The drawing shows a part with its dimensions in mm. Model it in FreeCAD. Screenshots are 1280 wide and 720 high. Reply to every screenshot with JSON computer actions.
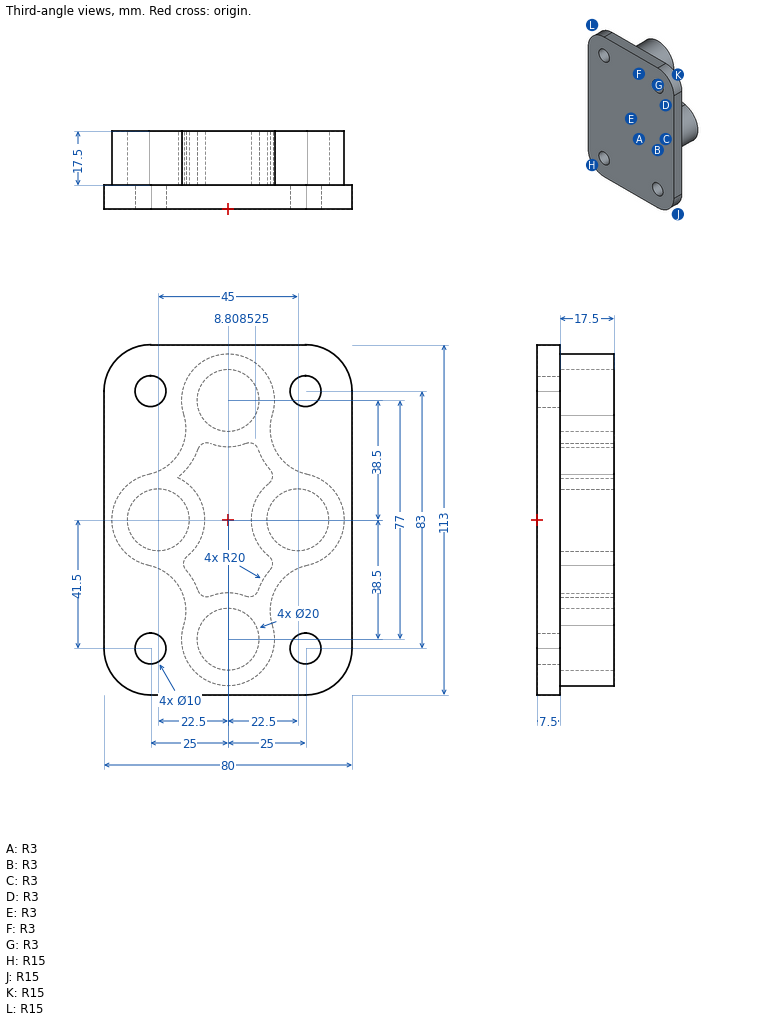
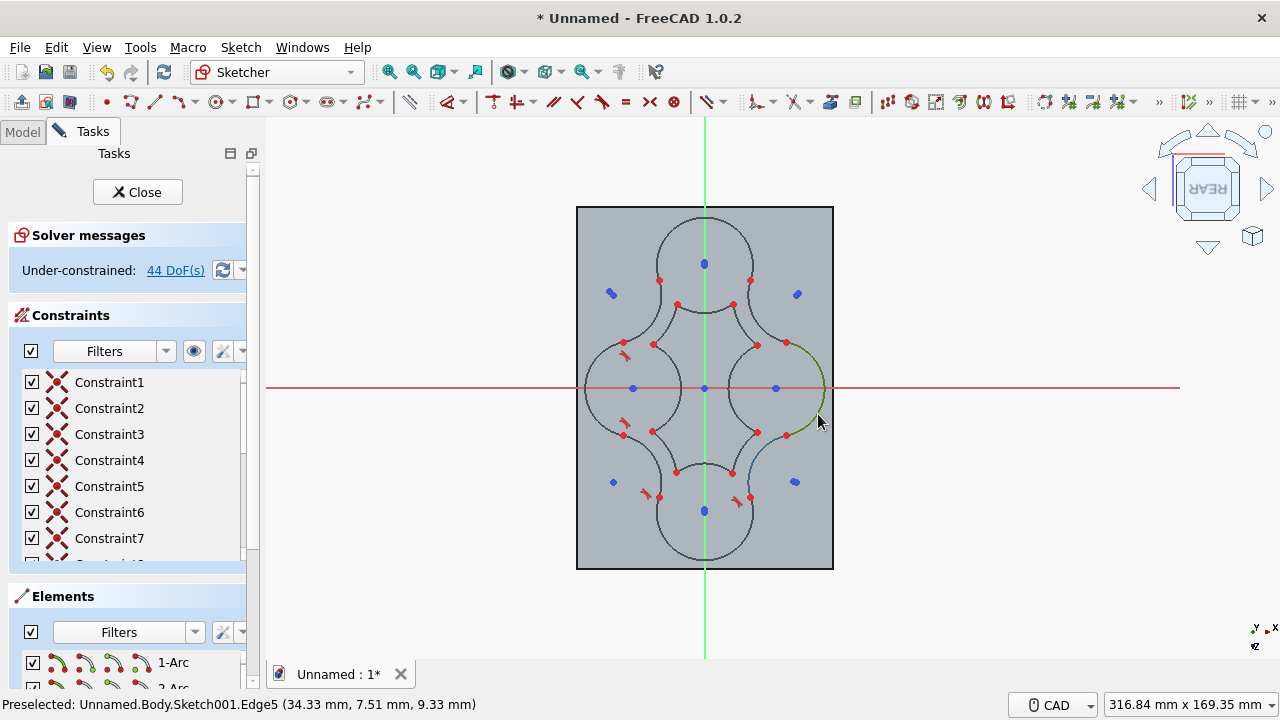
{"action": "key", "text": "t"}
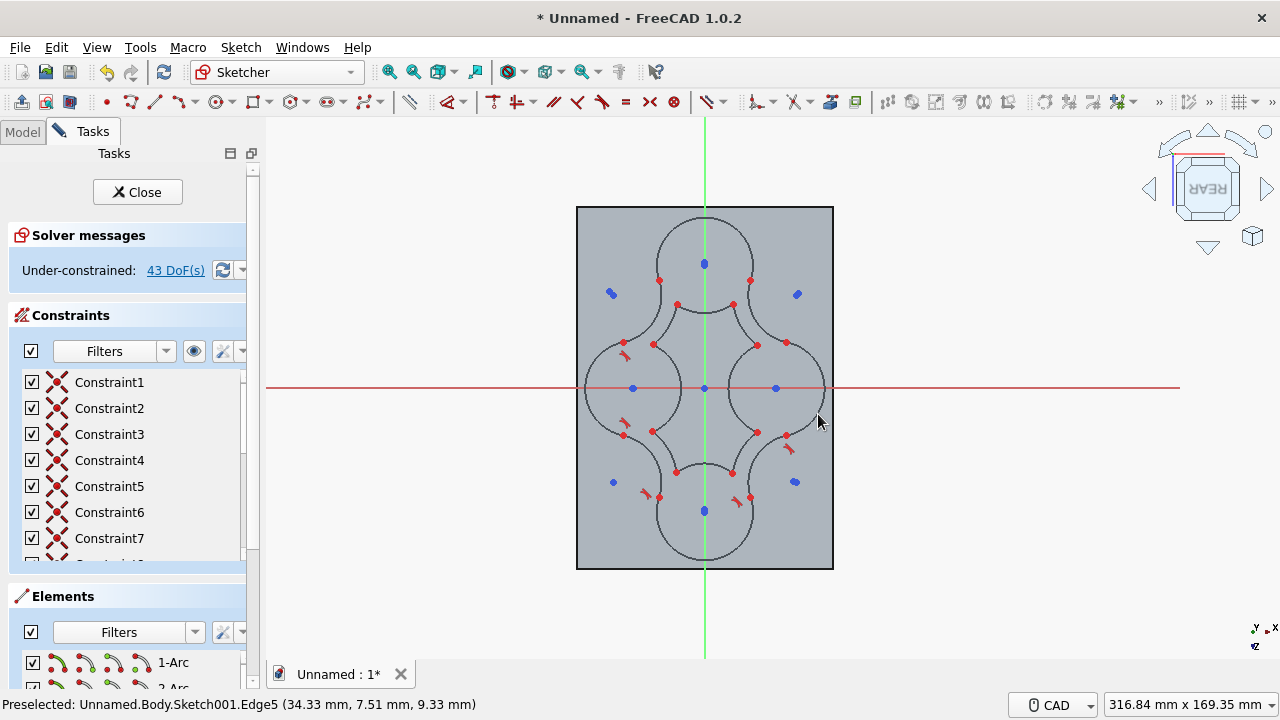
{"action": "left_click", "coordinate": [818, 414]}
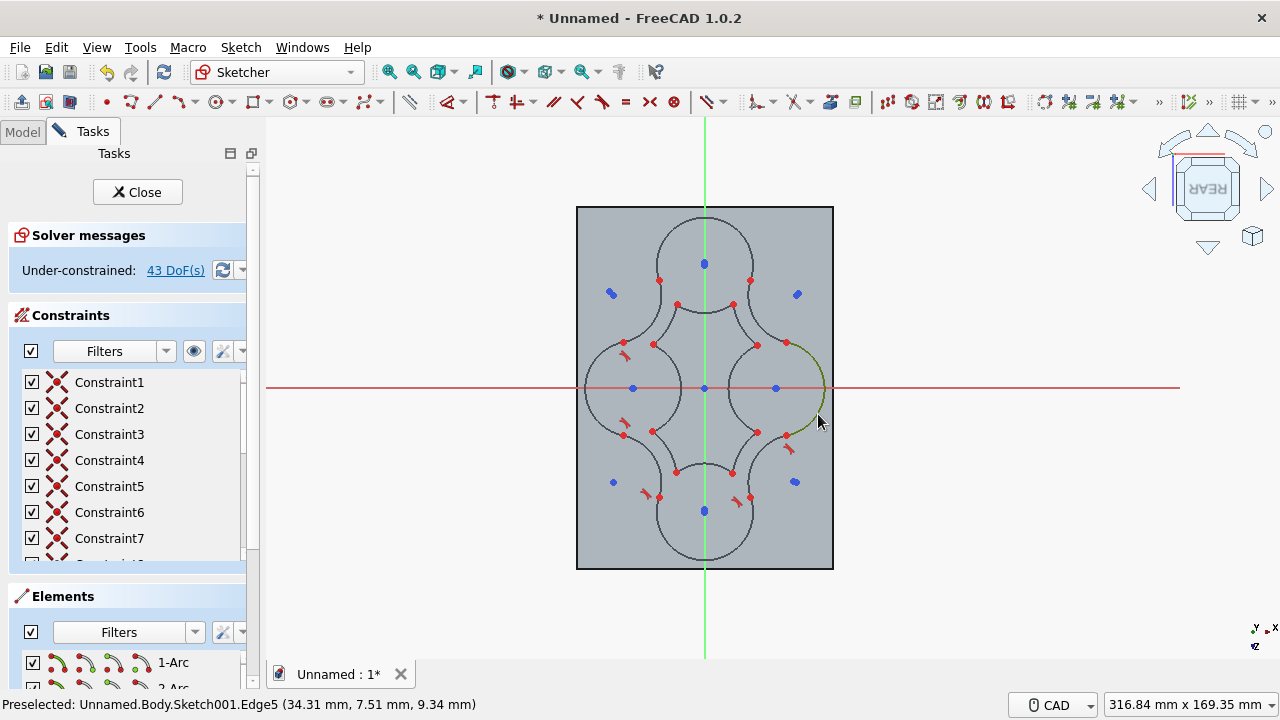
{"action": "left_click", "coordinate": [749, 304]}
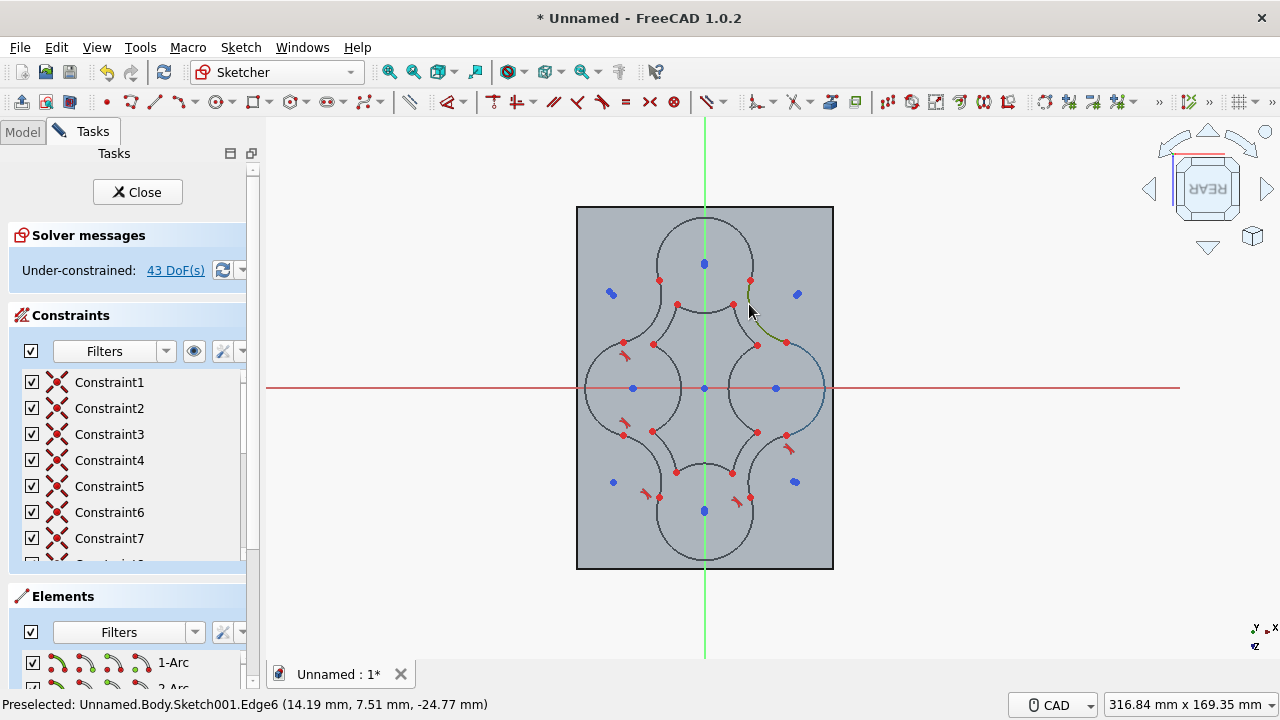
{"action": "key", "text": "t"}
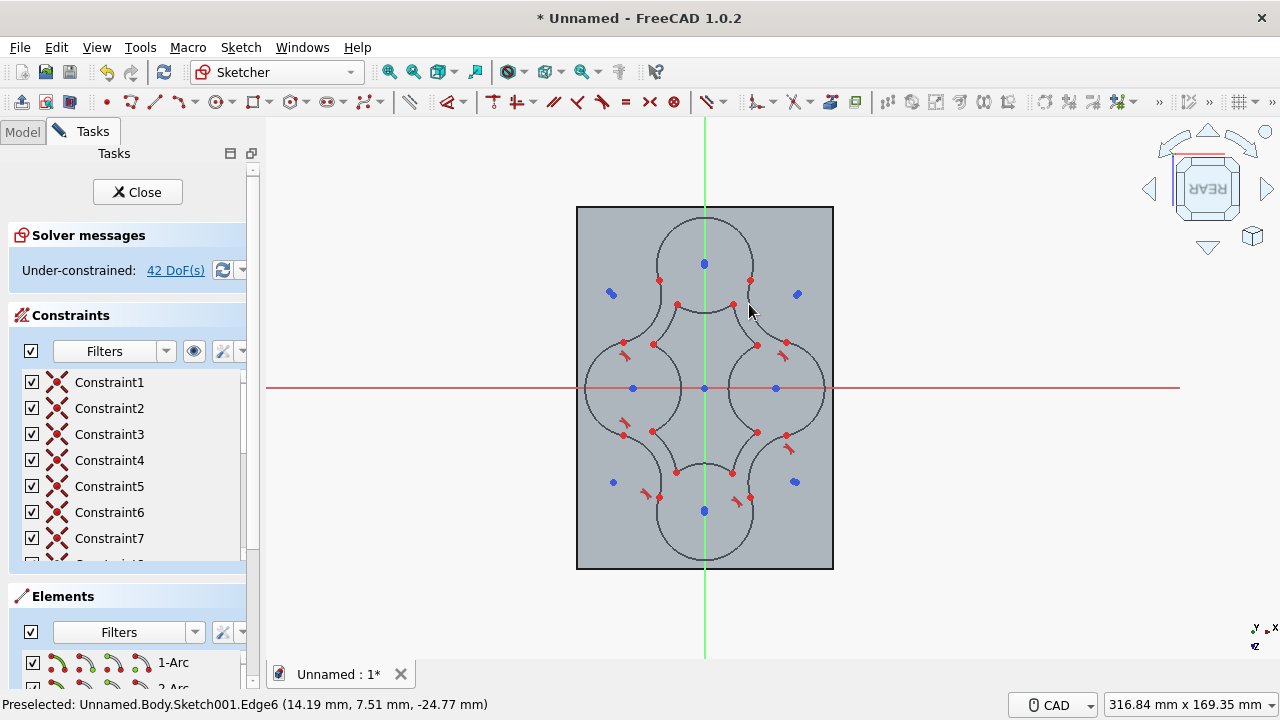
{"action": "left_click", "coordinate": [749, 304]}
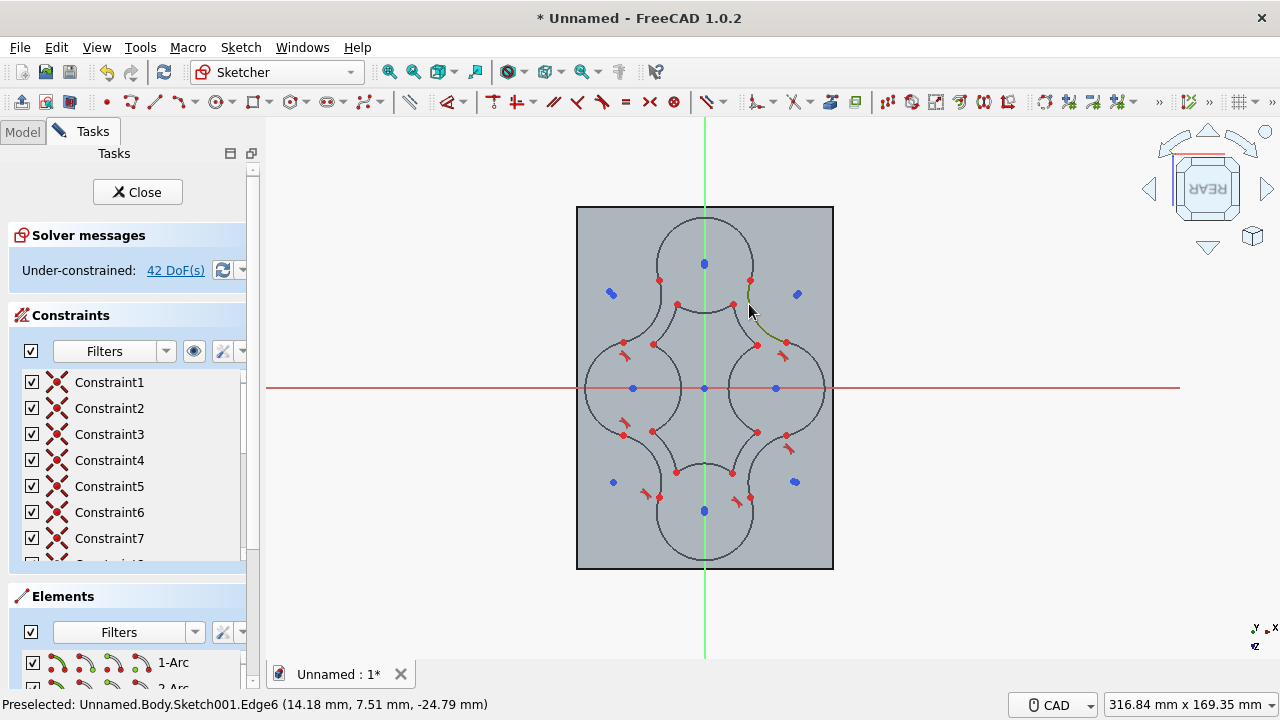
{"action": "left_click", "coordinate": [738, 230]}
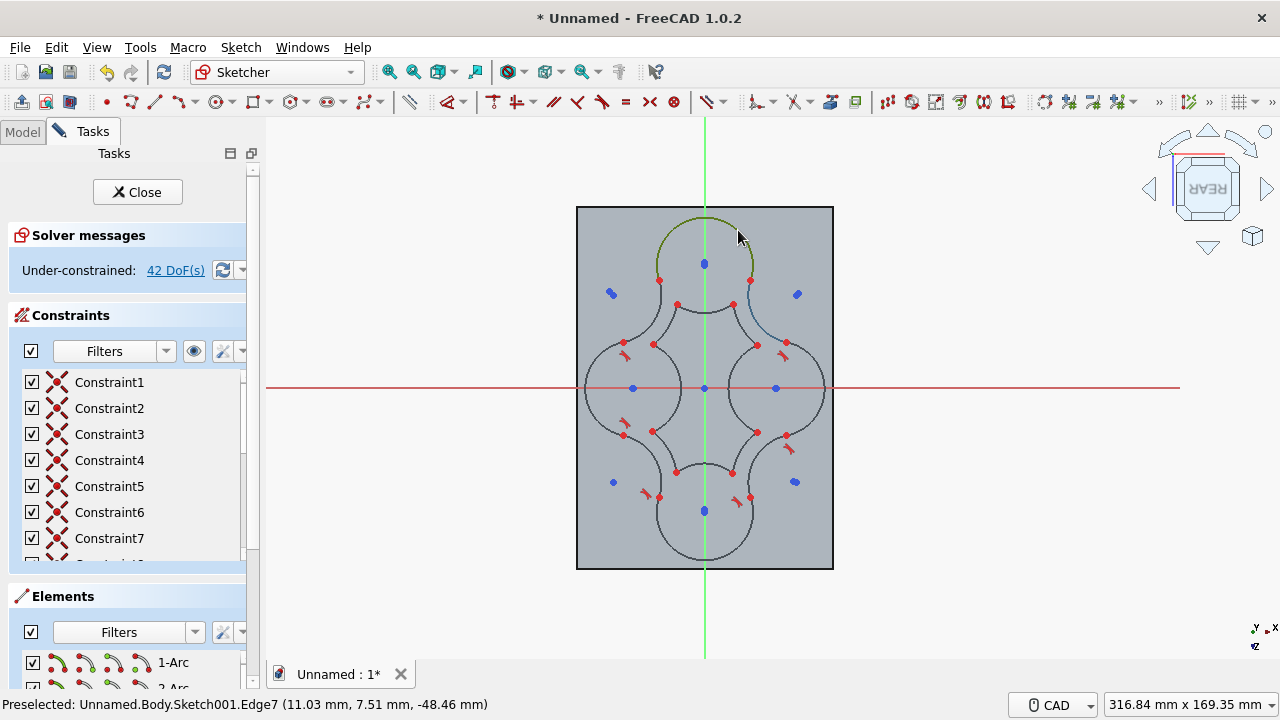
{"action": "left_click", "coordinate": [602, 102]}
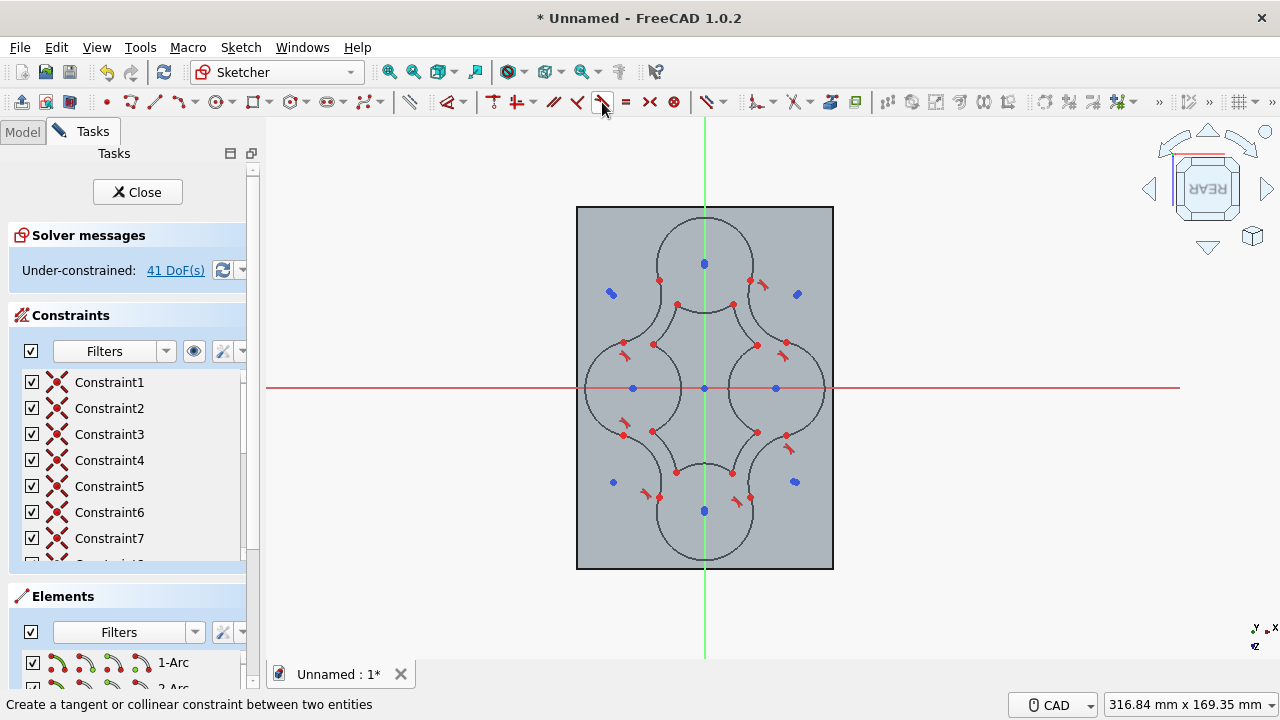
{"action": "left_click", "coordinate": [738, 231]}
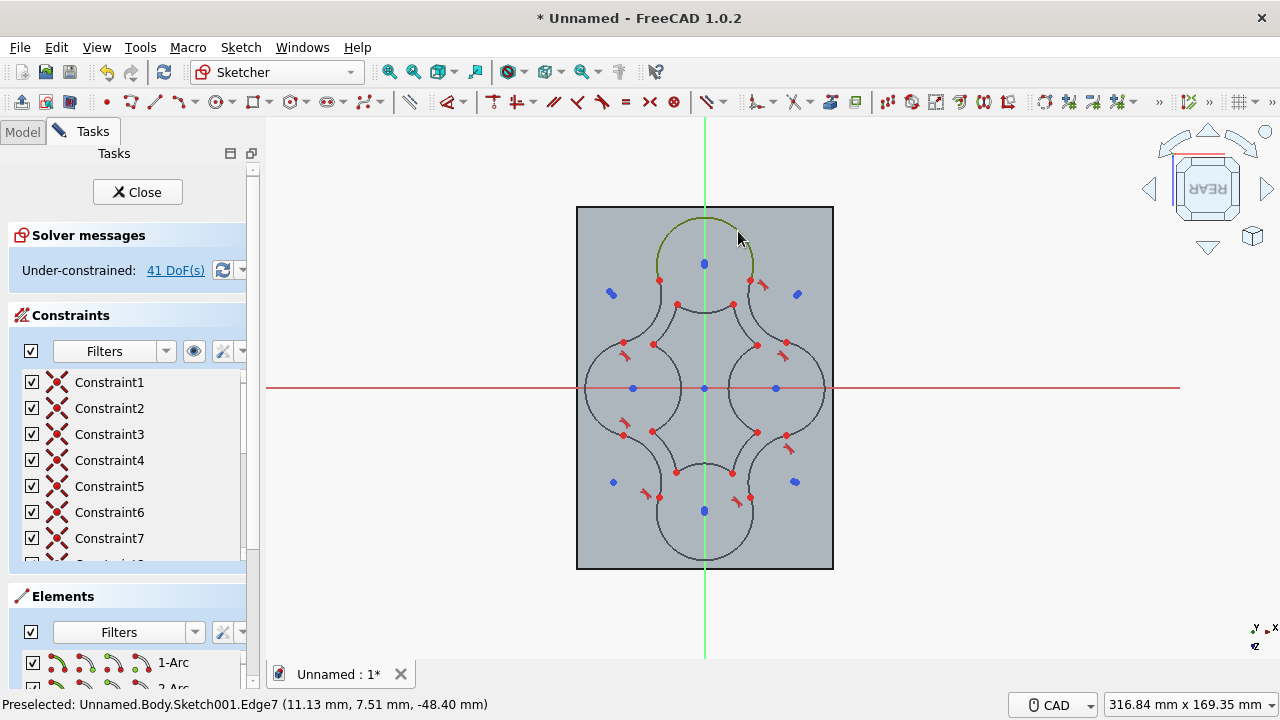
{"action": "left_click", "coordinate": [645, 332]}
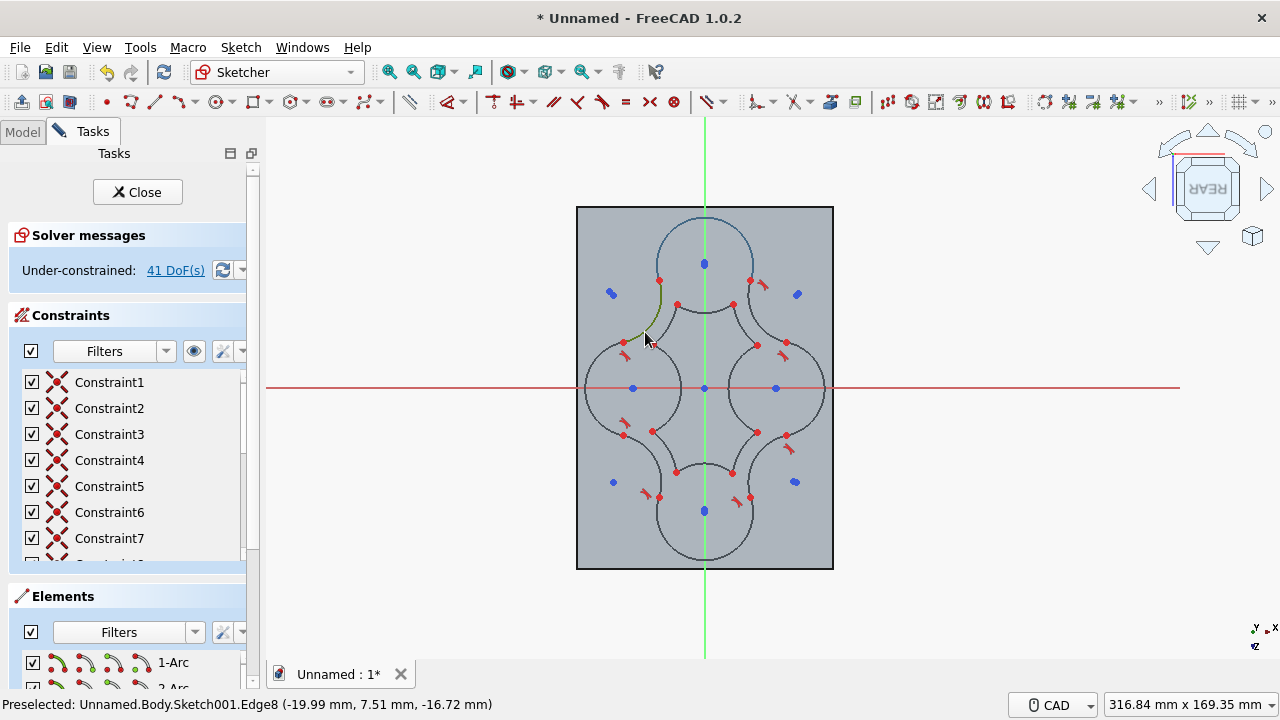
{"action": "key", "text": "t"}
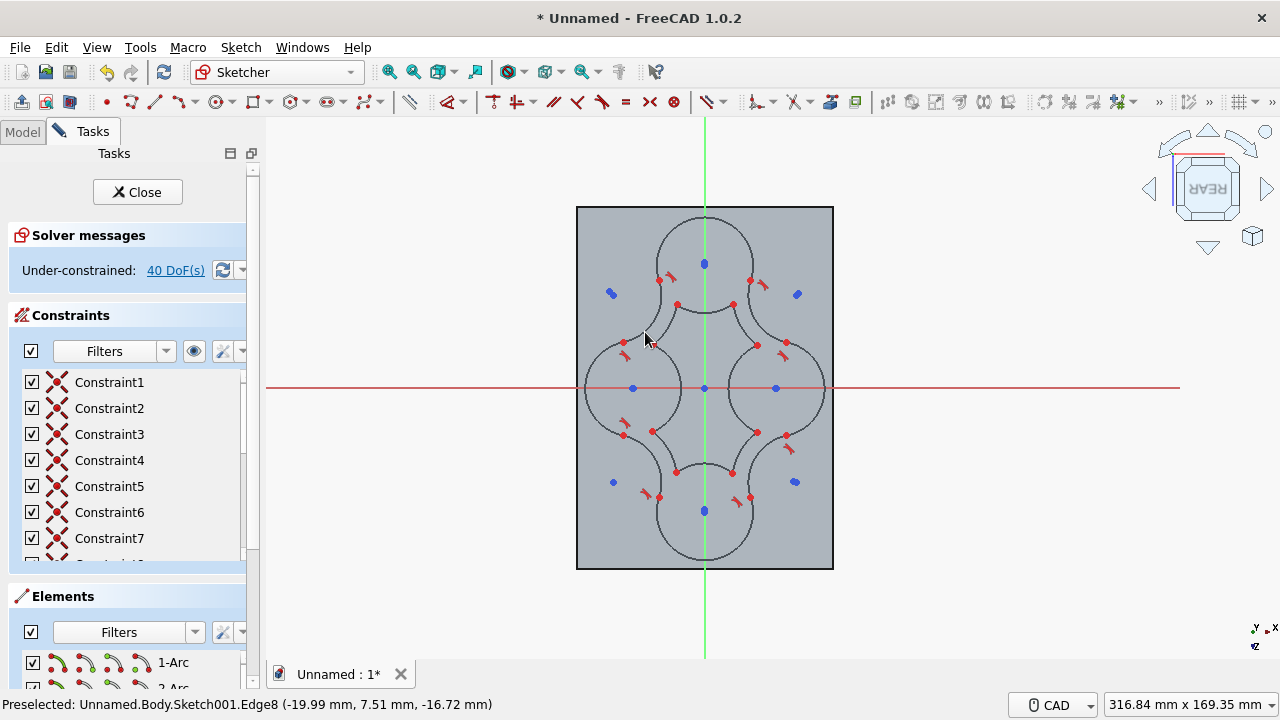
{"action": "left_click", "coordinate": [818, 414]}